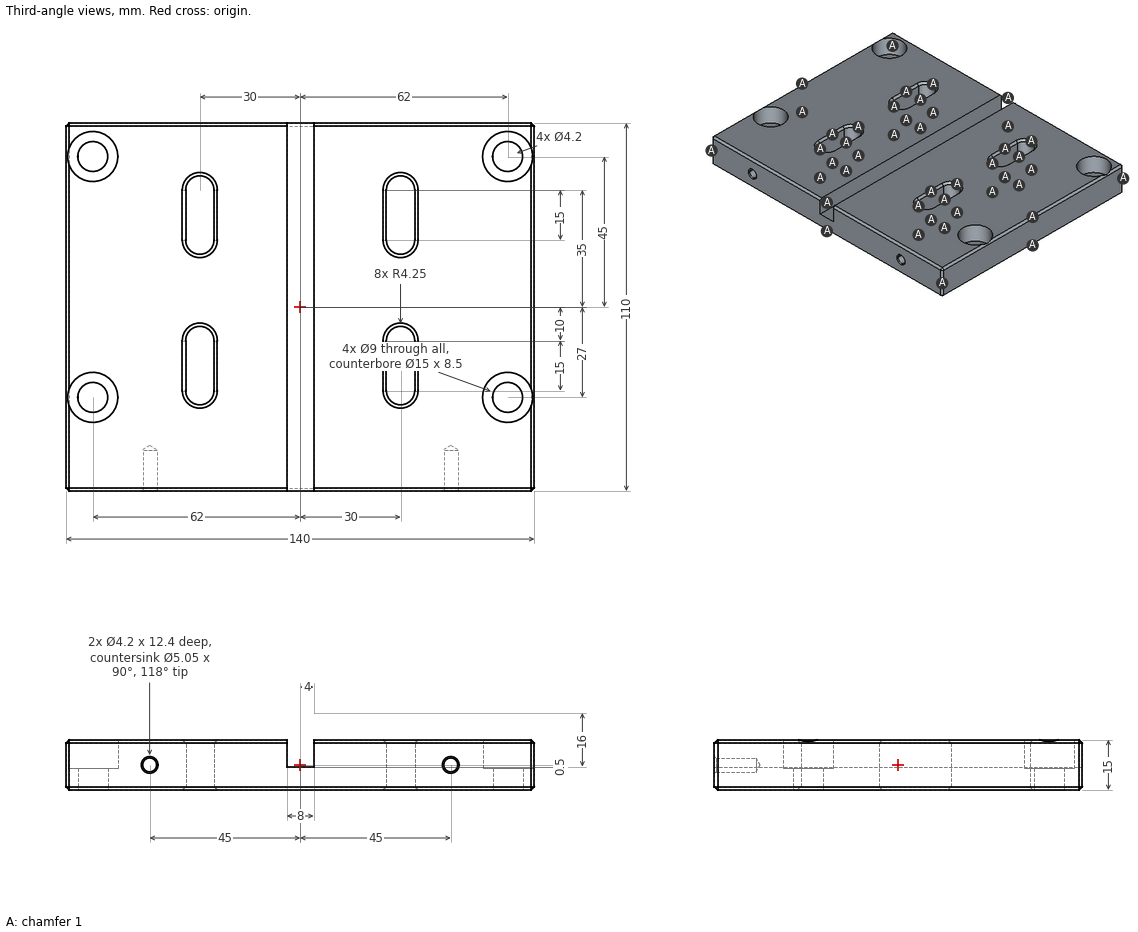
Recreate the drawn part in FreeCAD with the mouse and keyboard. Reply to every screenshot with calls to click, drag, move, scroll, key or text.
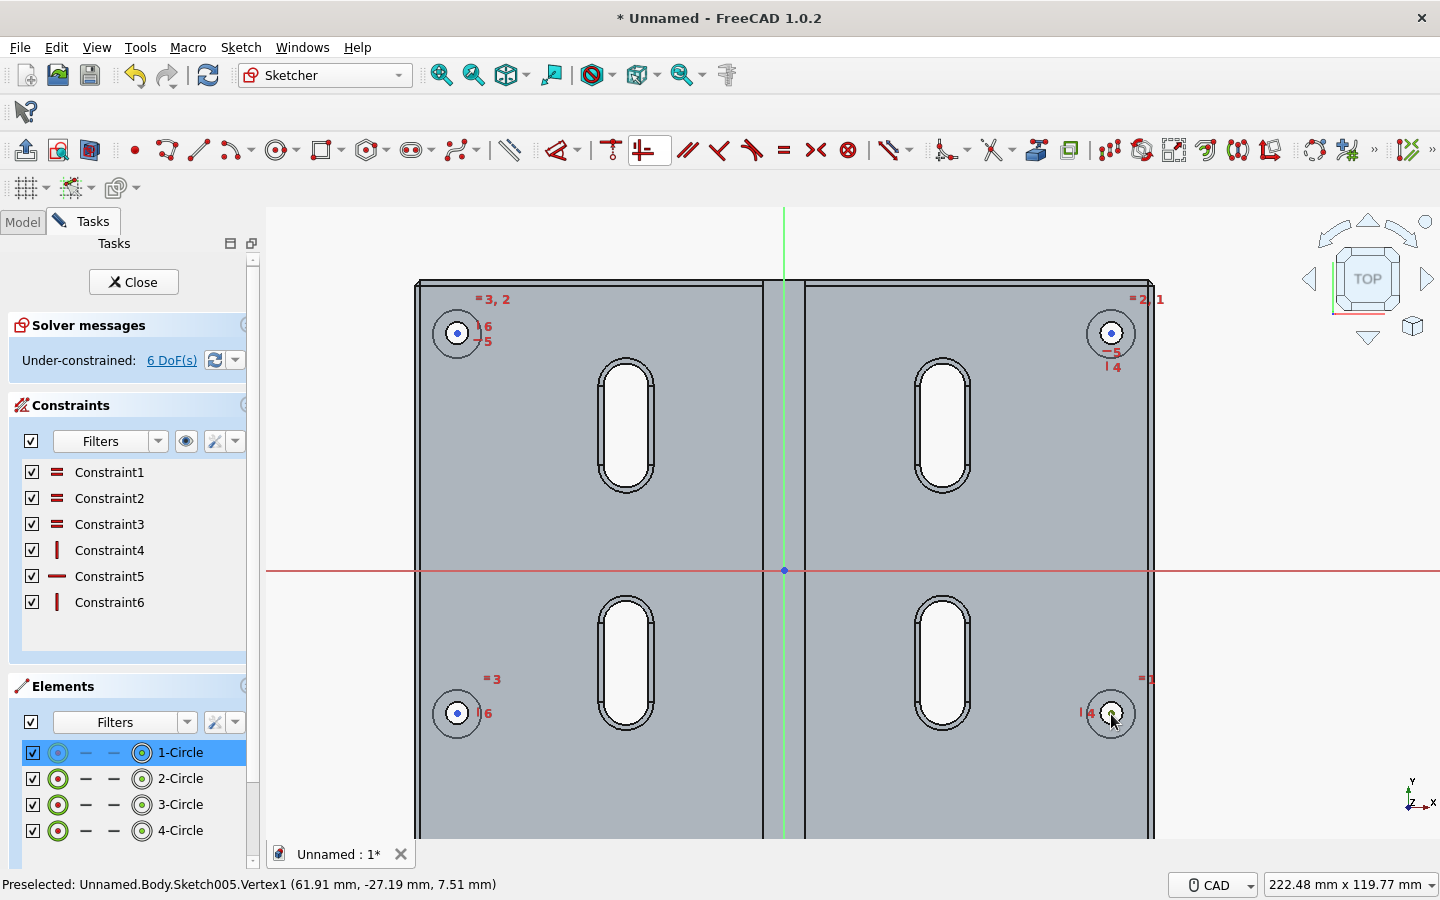
click(457, 714)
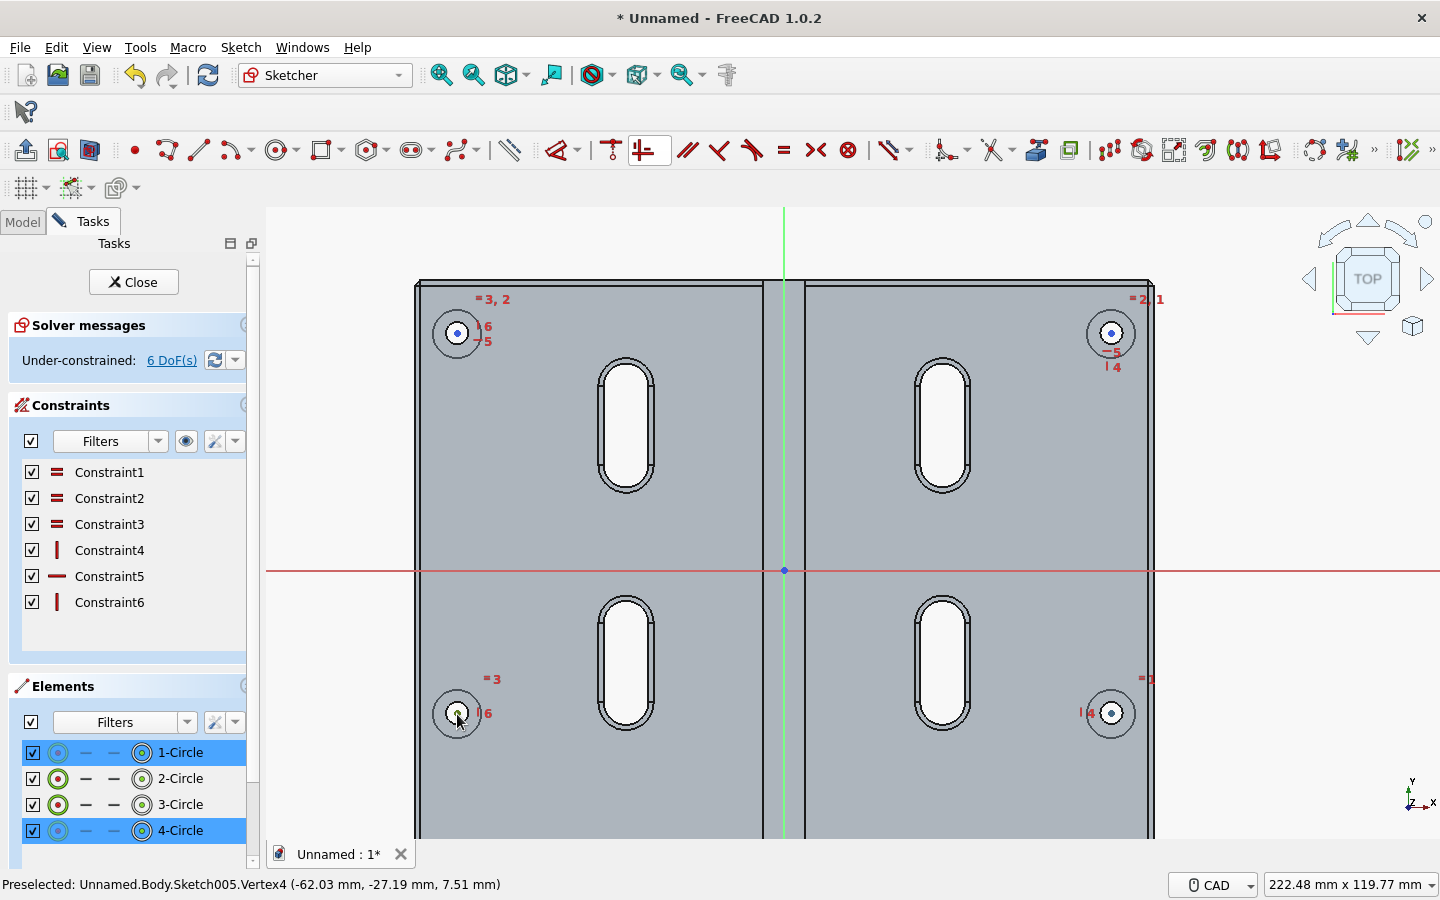
key(h)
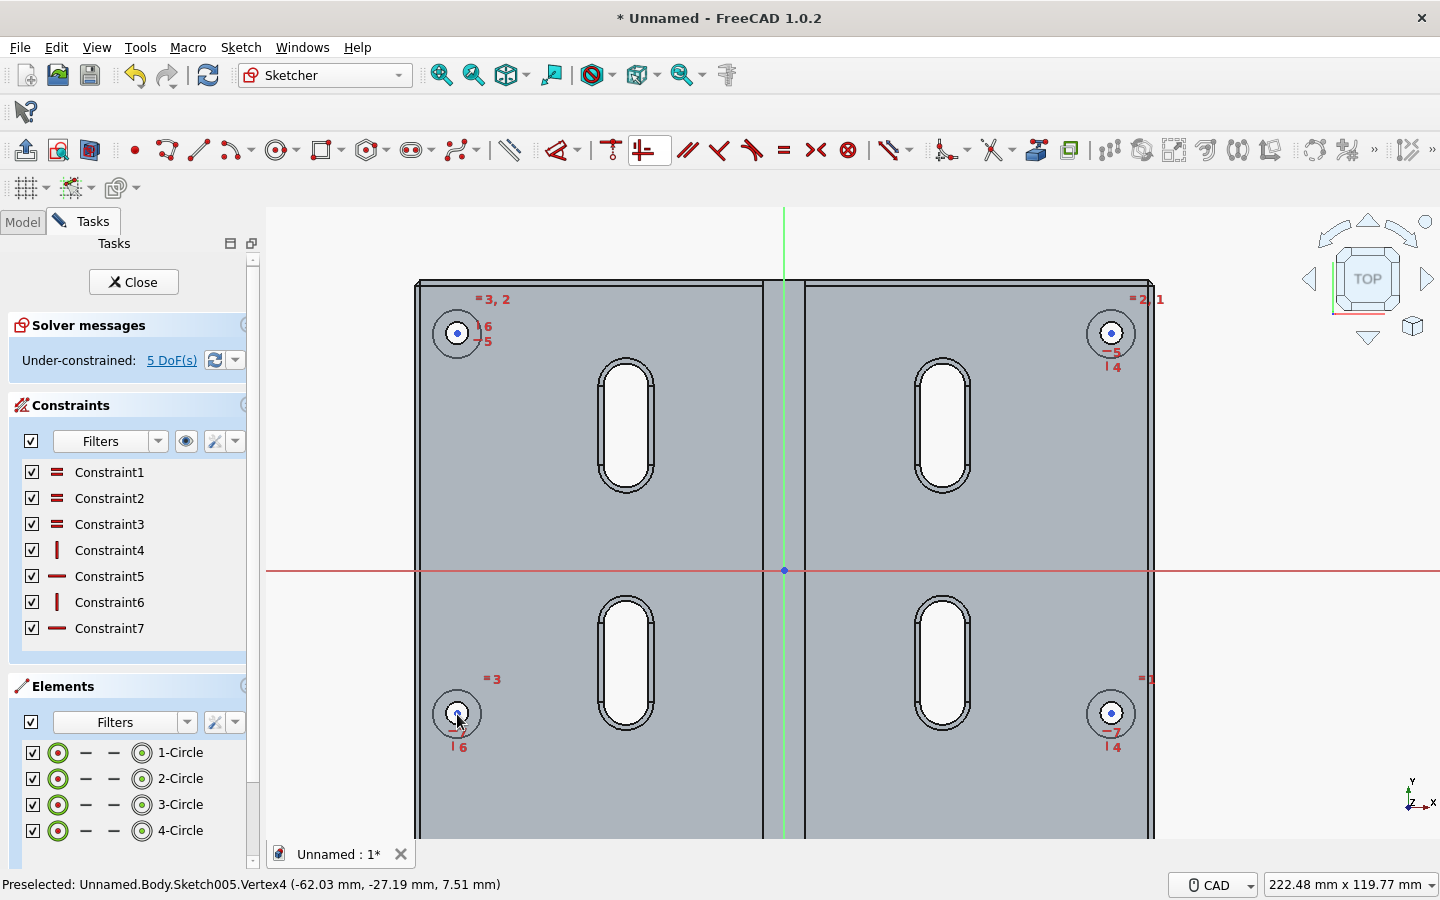
key(d)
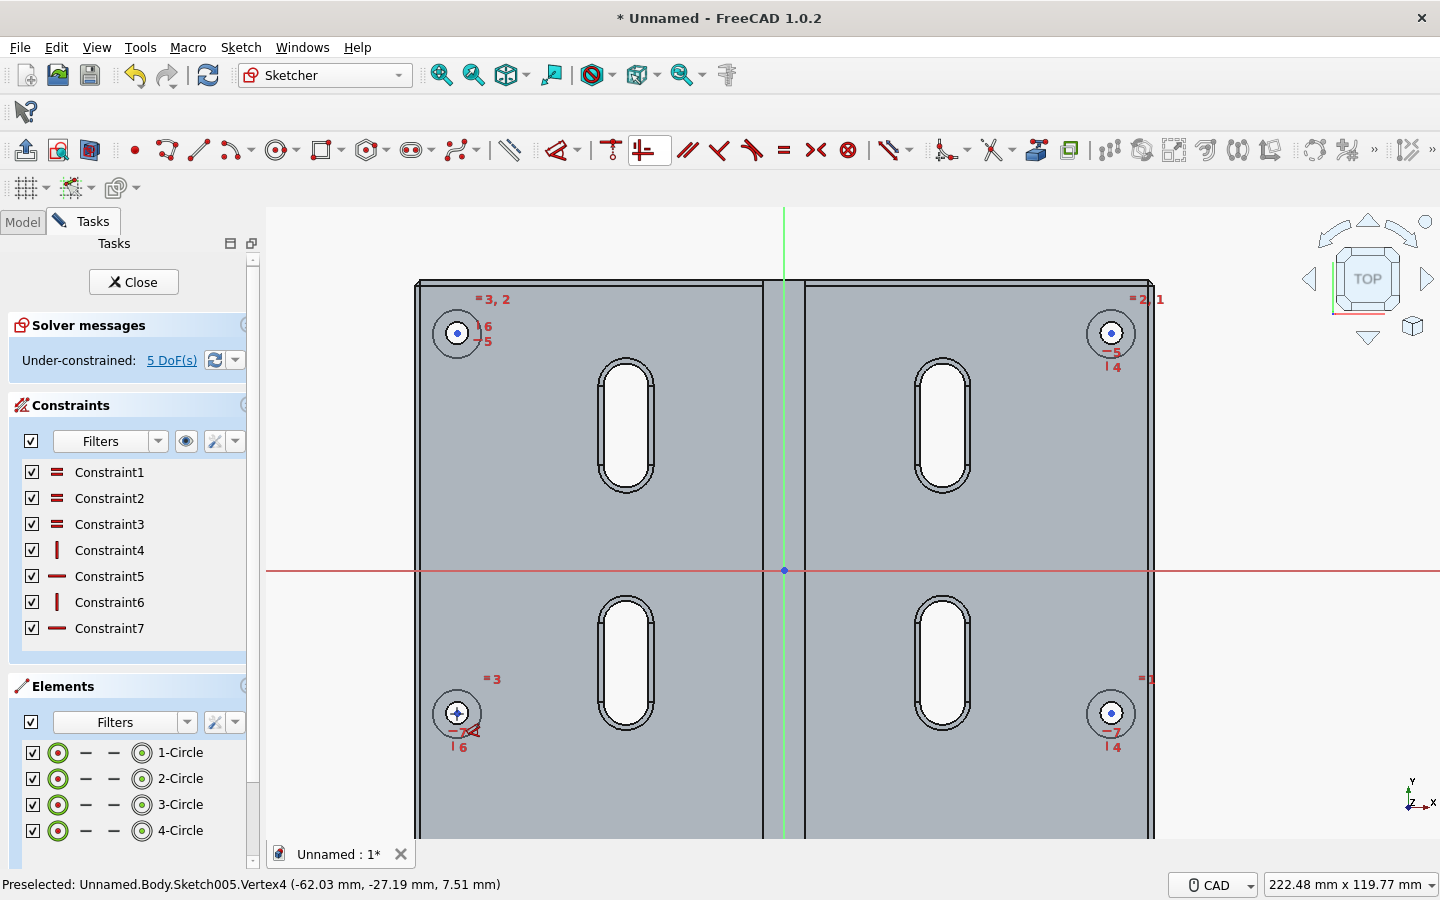
click(1128, 697)
click(1151, 674)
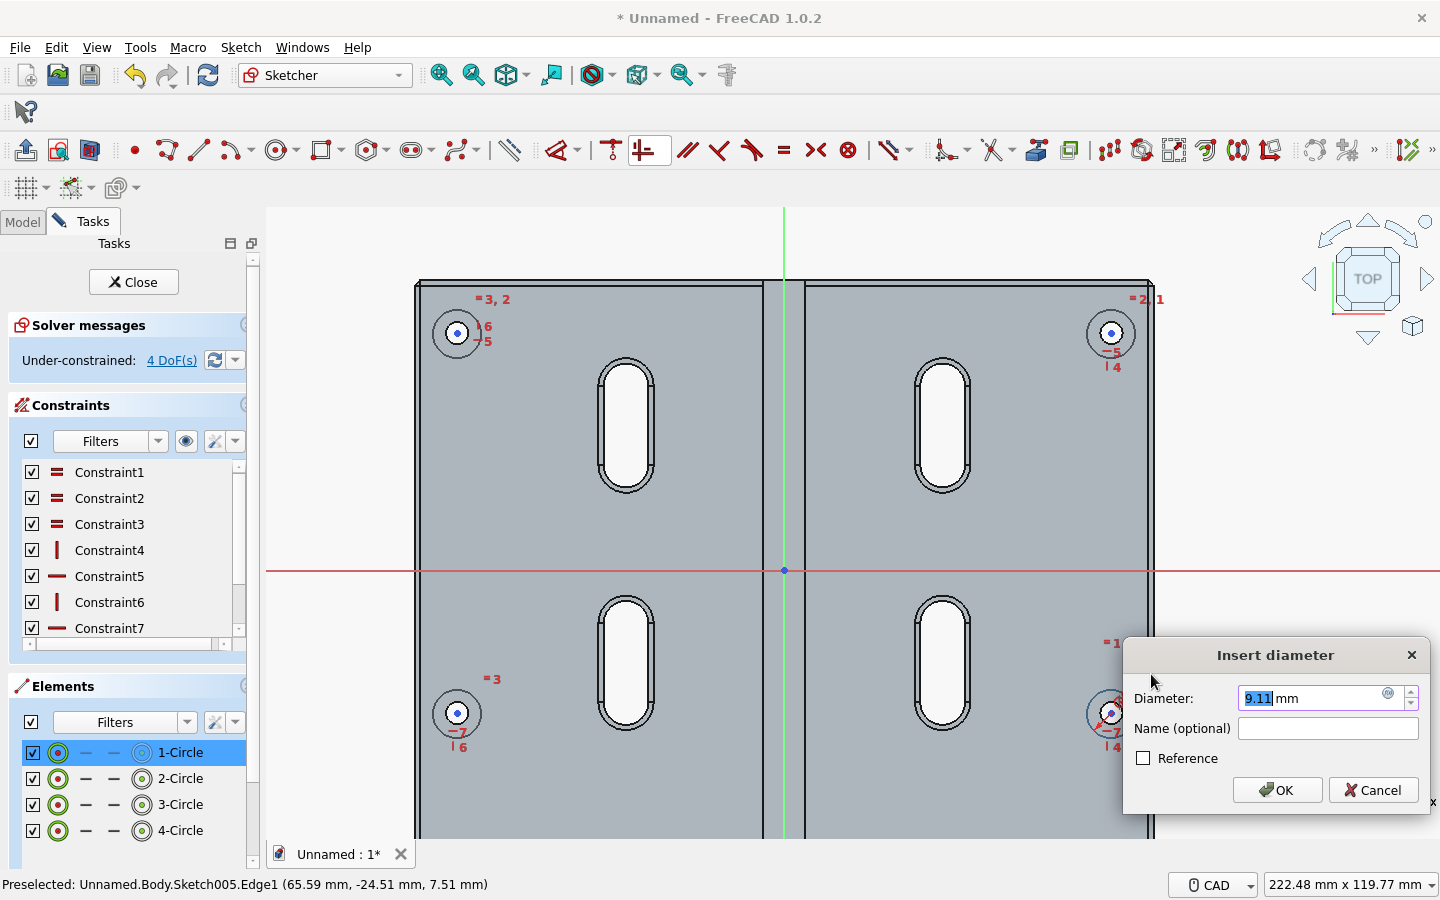
text(9)
key(Return)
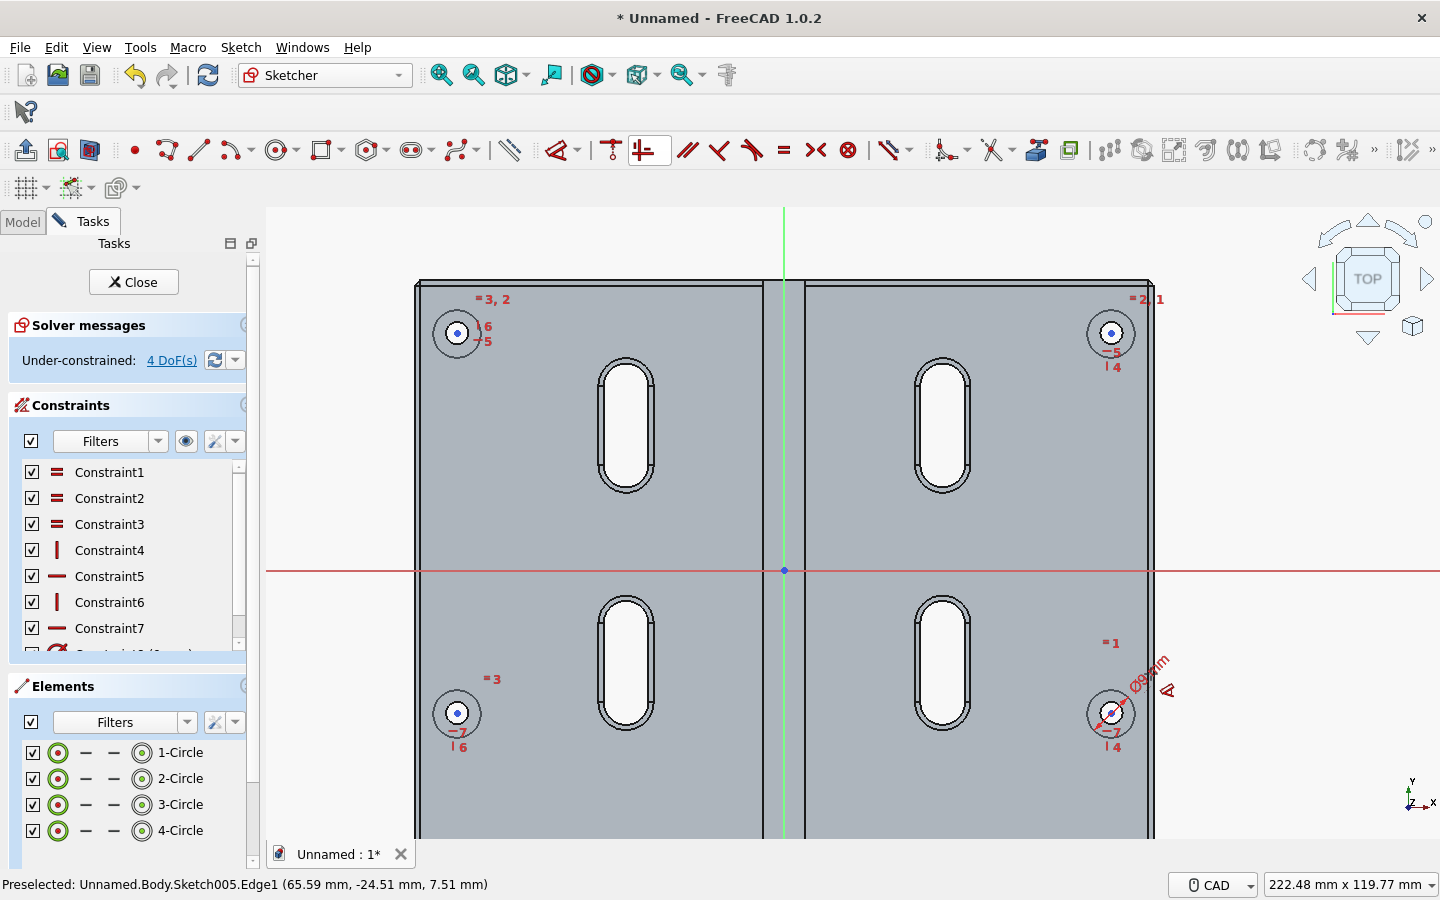
click(1111, 714)
click(948, 748)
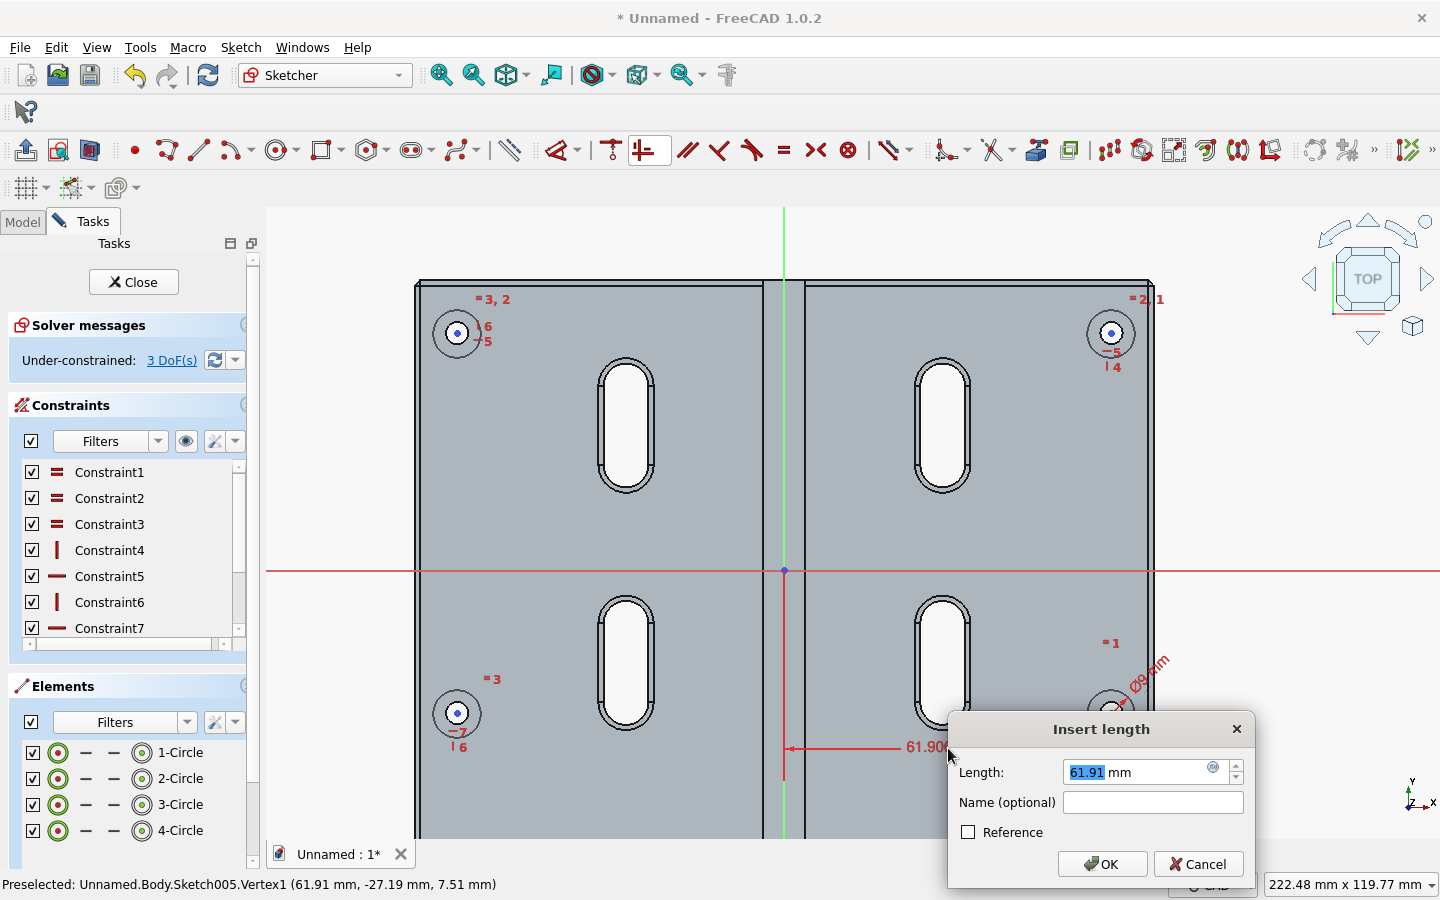
text(62)
key(Return)